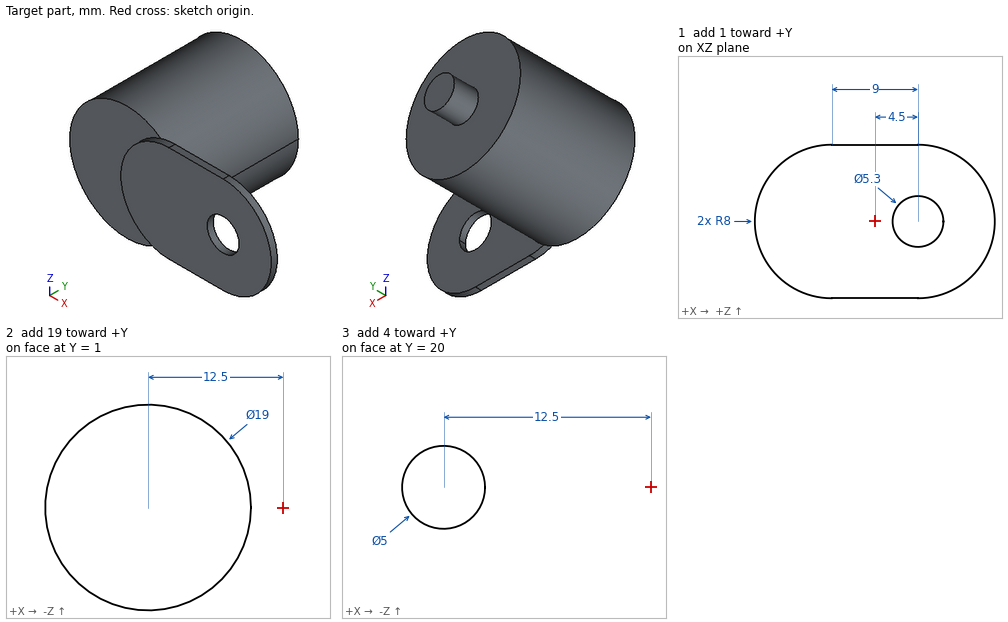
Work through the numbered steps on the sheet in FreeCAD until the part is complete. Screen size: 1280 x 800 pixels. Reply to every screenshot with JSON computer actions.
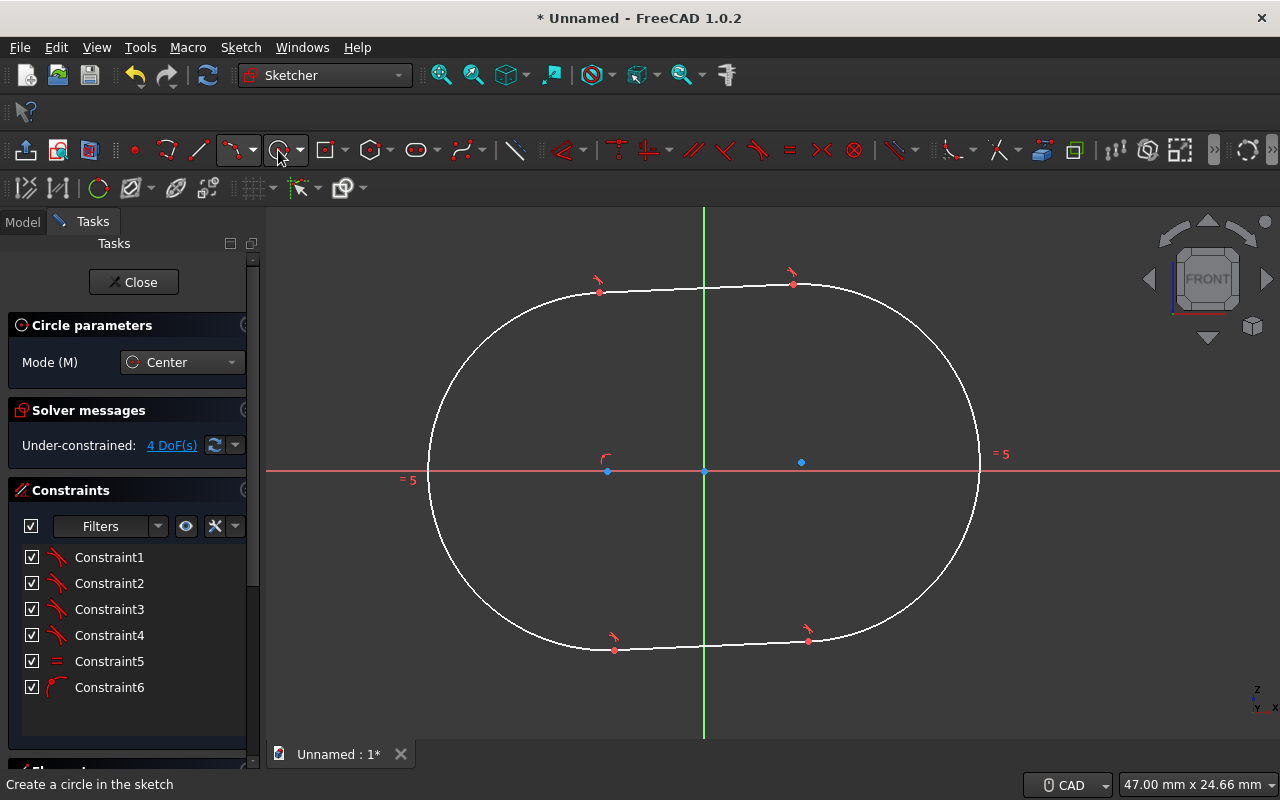
{"action": "left_click", "coordinate": [801, 463]}
{"action": "left_click", "coordinate": [842, 431]}
{"action": "key", "text": "Escape"}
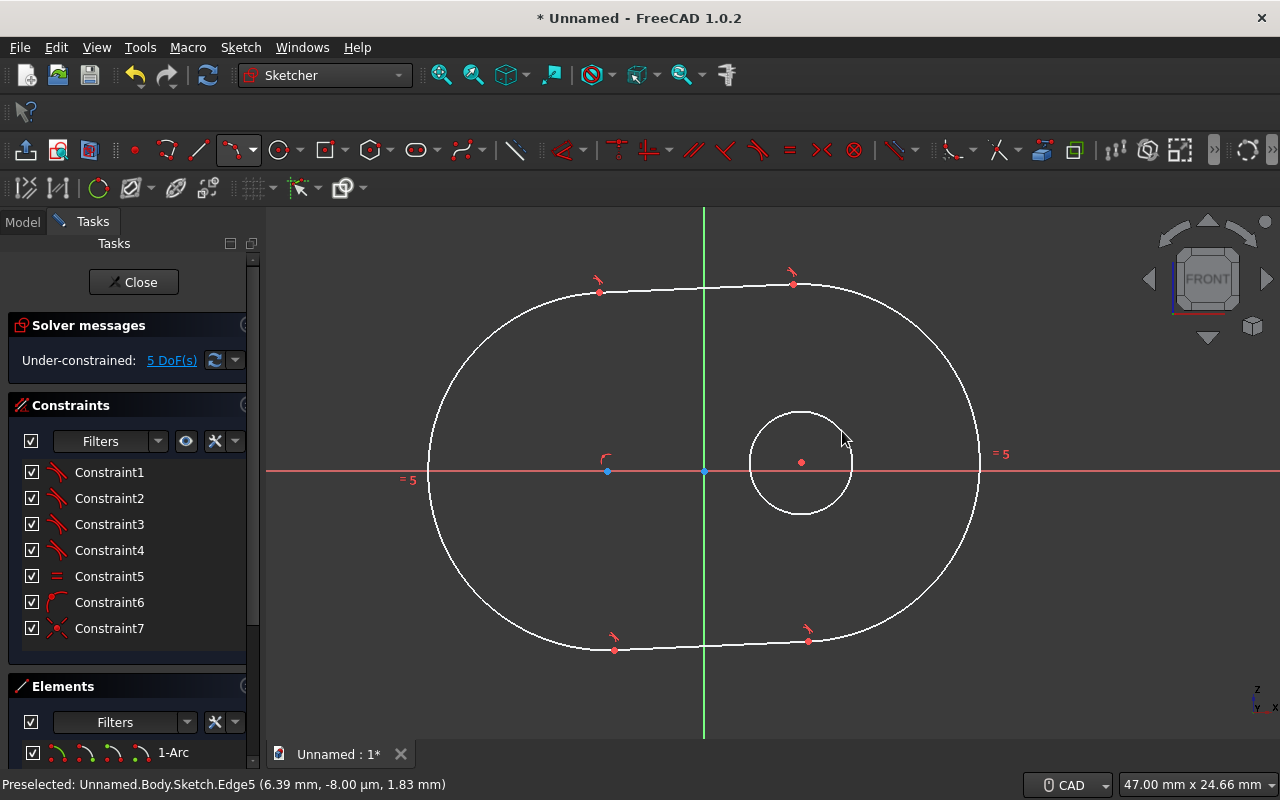
{"action": "left_click", "coordinate": [657, 290]}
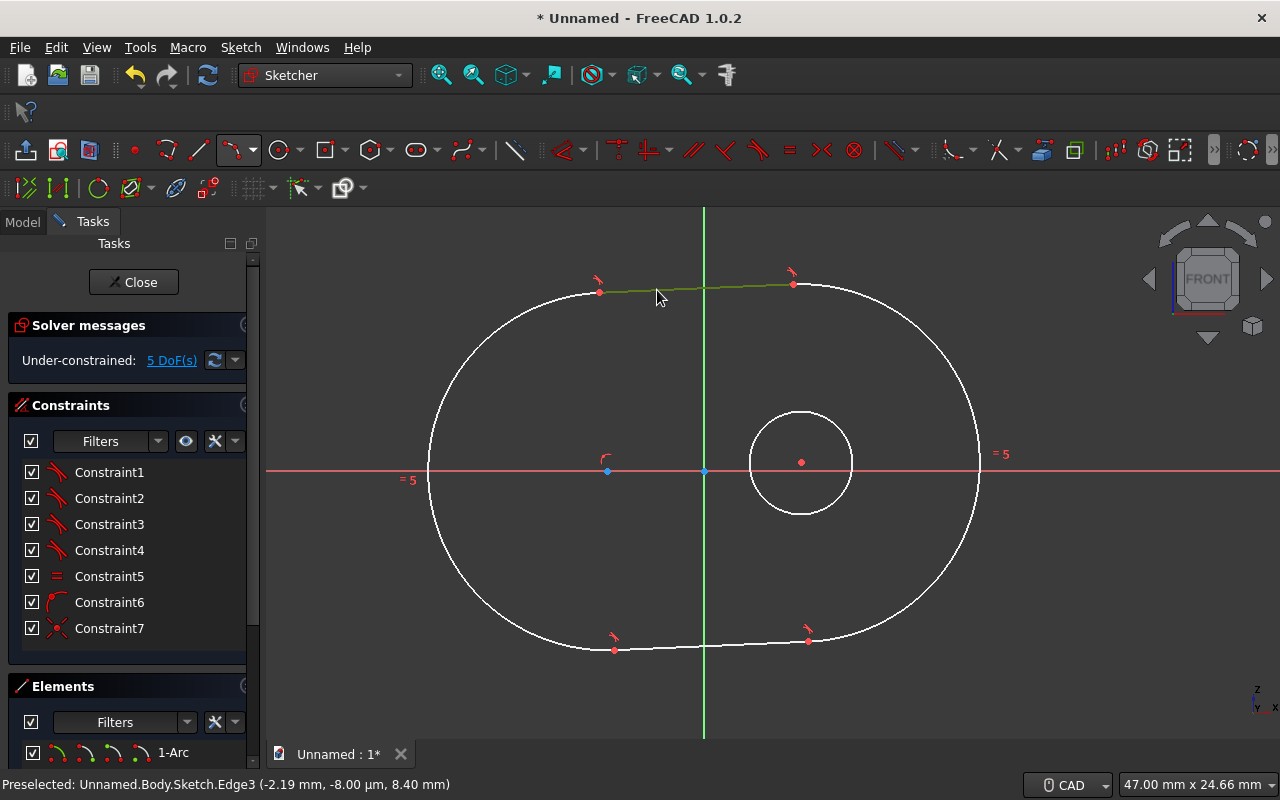
{"action": "key", "text": "h"}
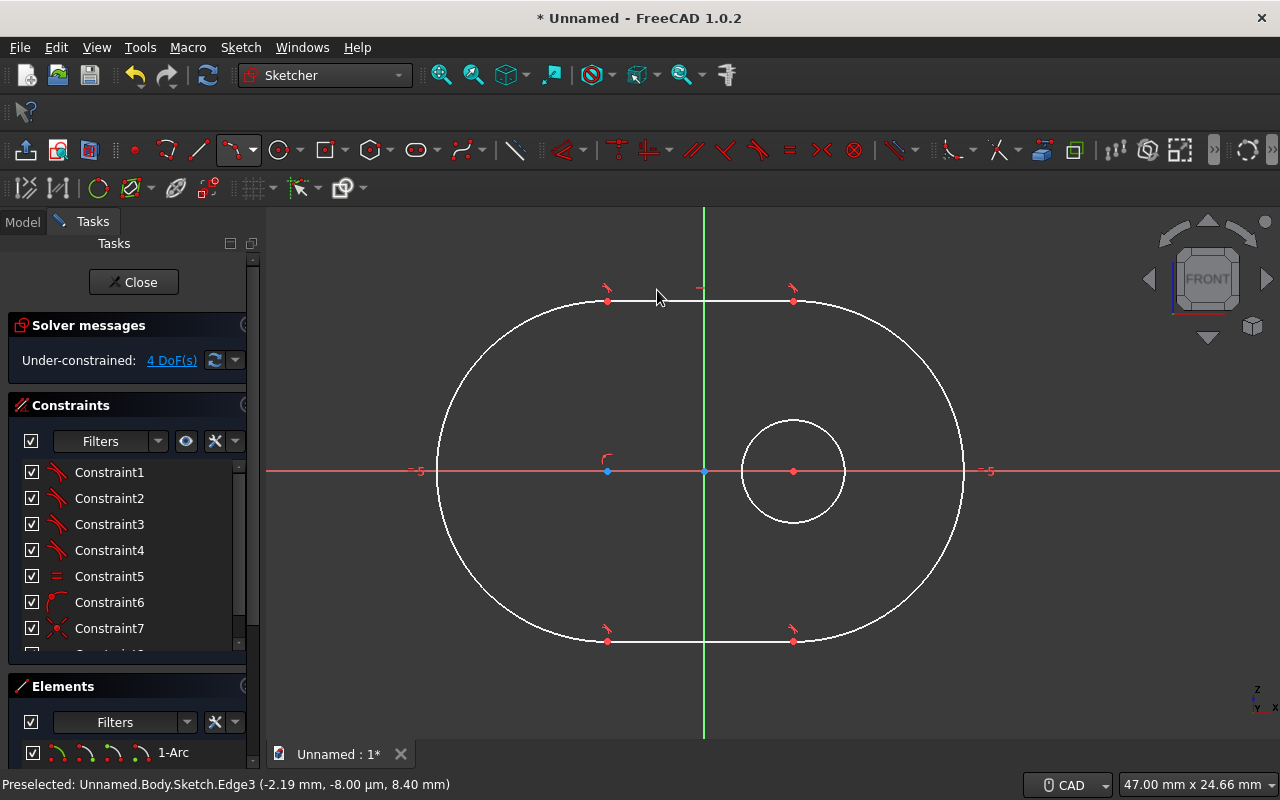
{"action": "left_click", "coordinate": [562, 150]}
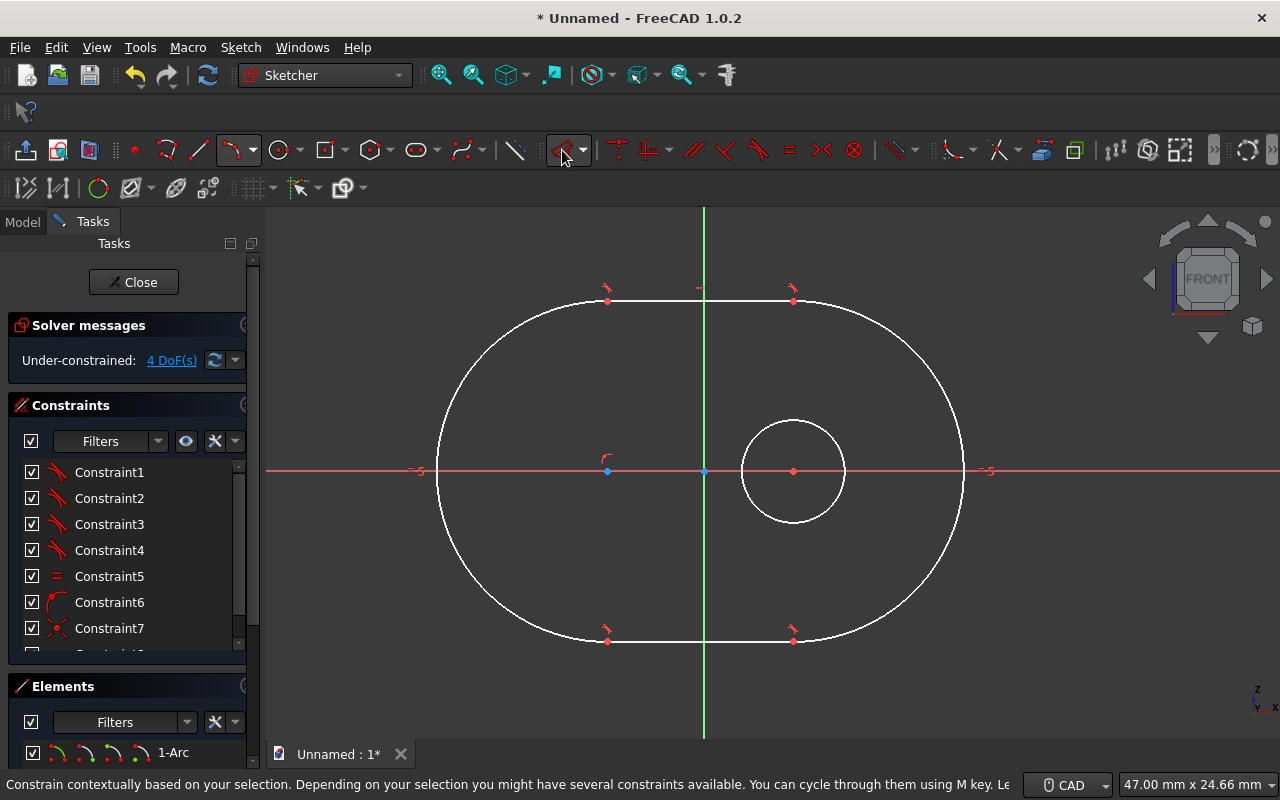
{"action": "left_click", "coordinate": [469, 371]}
{"action": "left_click", "coordinate": [443, 352]}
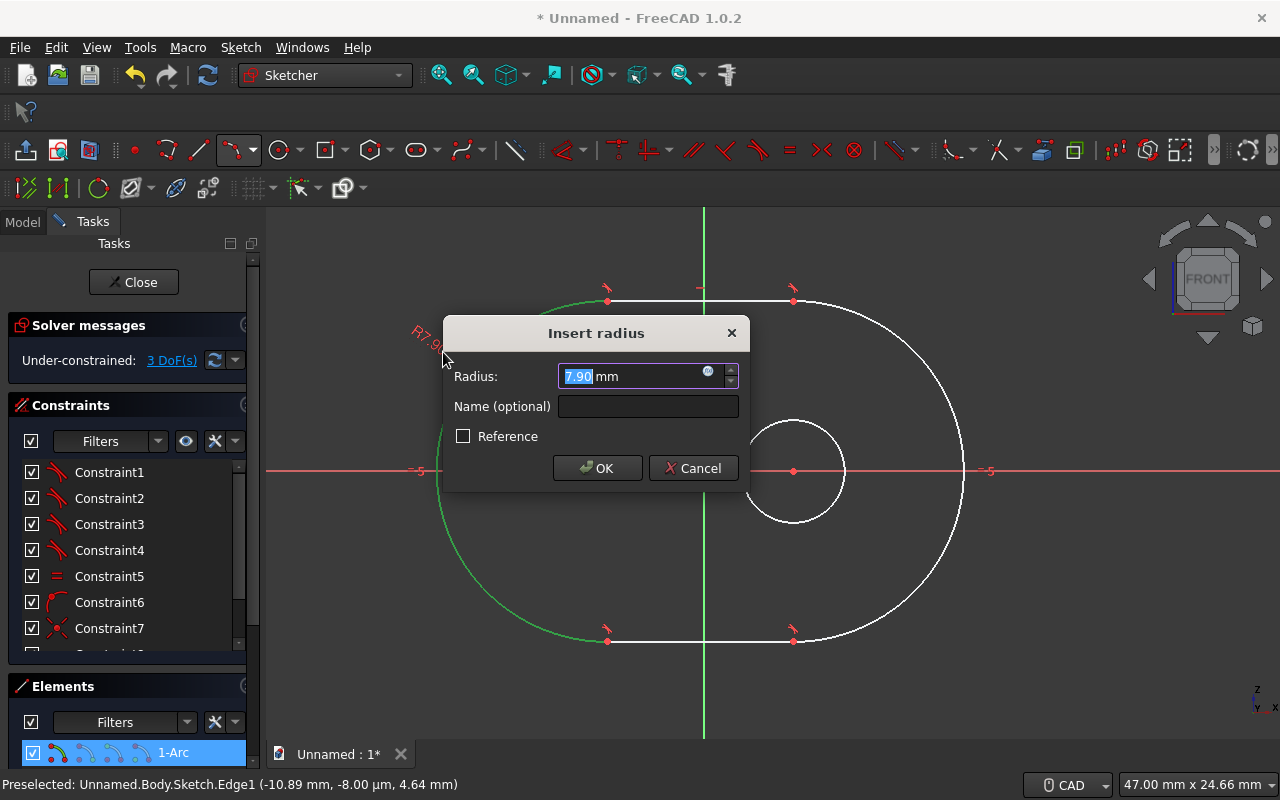
{"action": "type", "text": "8"}
{"action": "key", "text": "Return"}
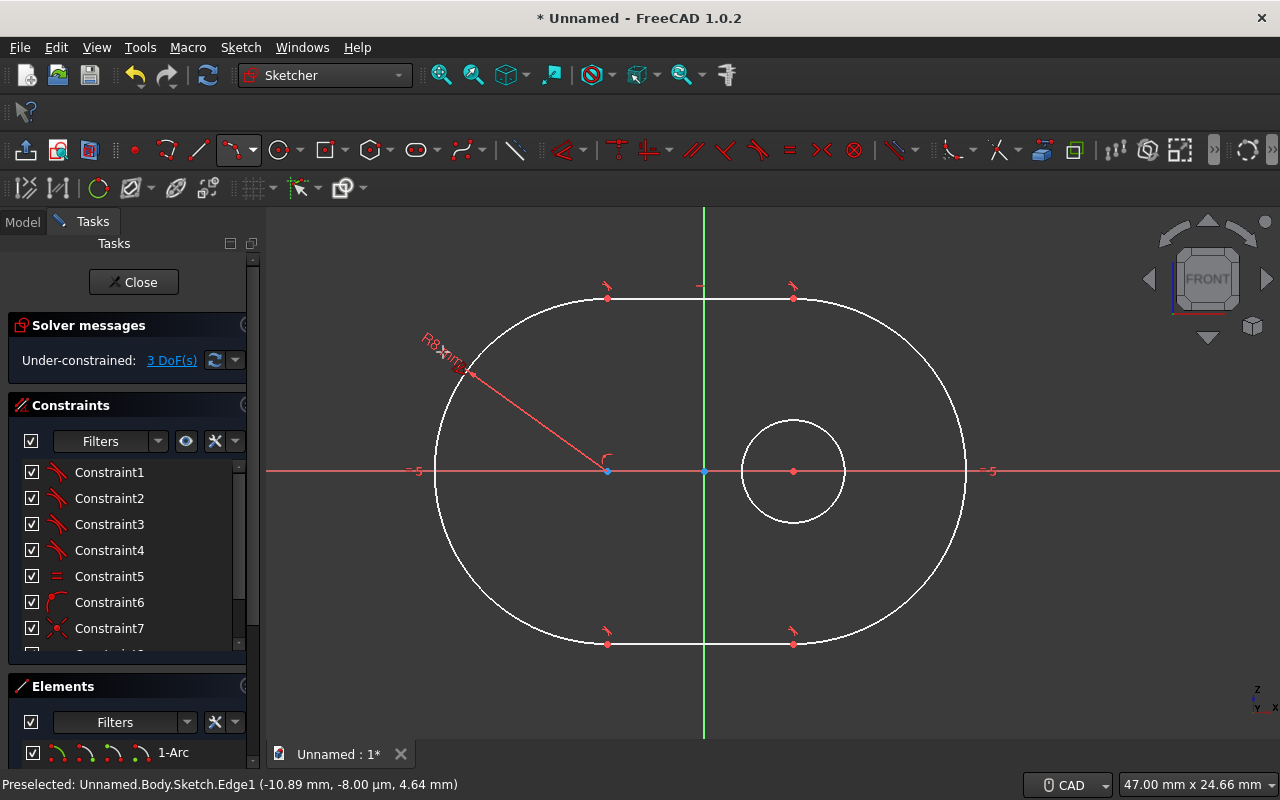
{"action": "left_click", "coordinate": [830, 435]}
{"action": "left_click", "coordinate": [853, 412]}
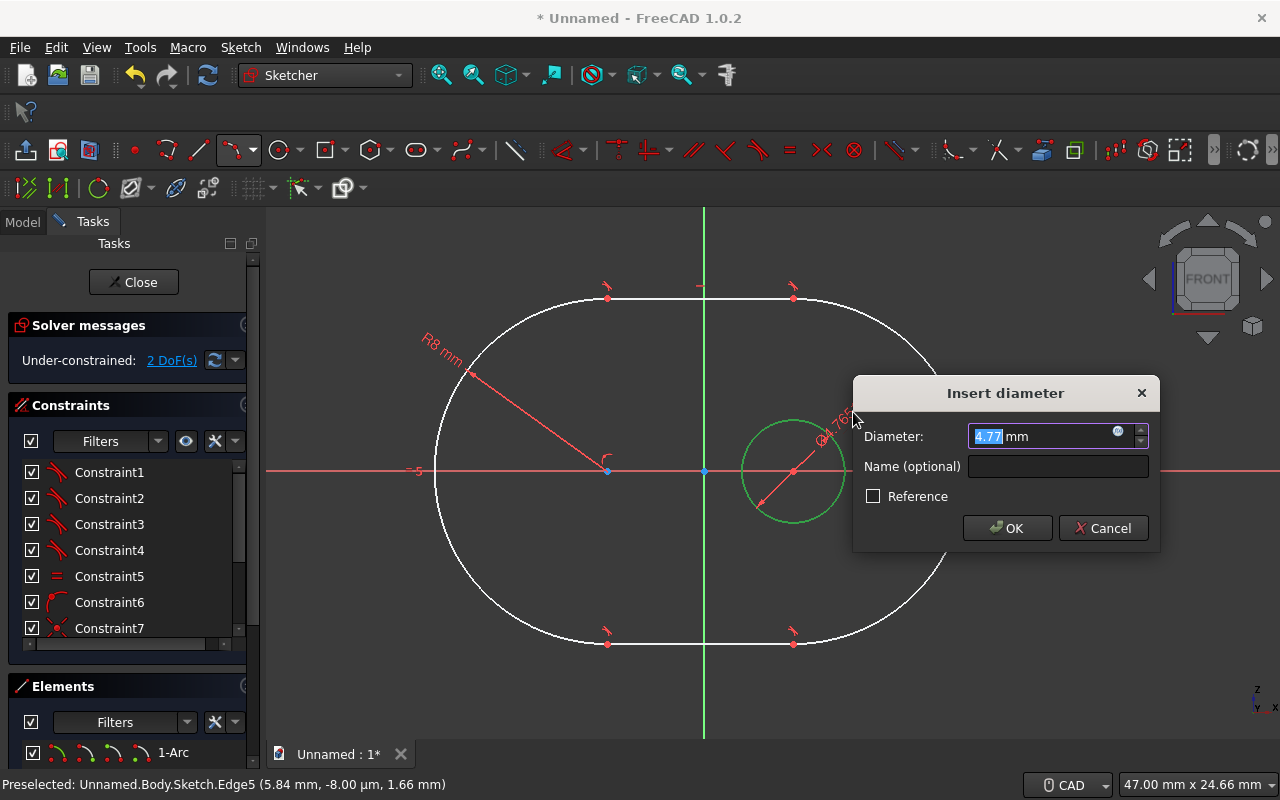
{"action": "type", "text": "5.3"}
{"action": "key", "text": "Return"}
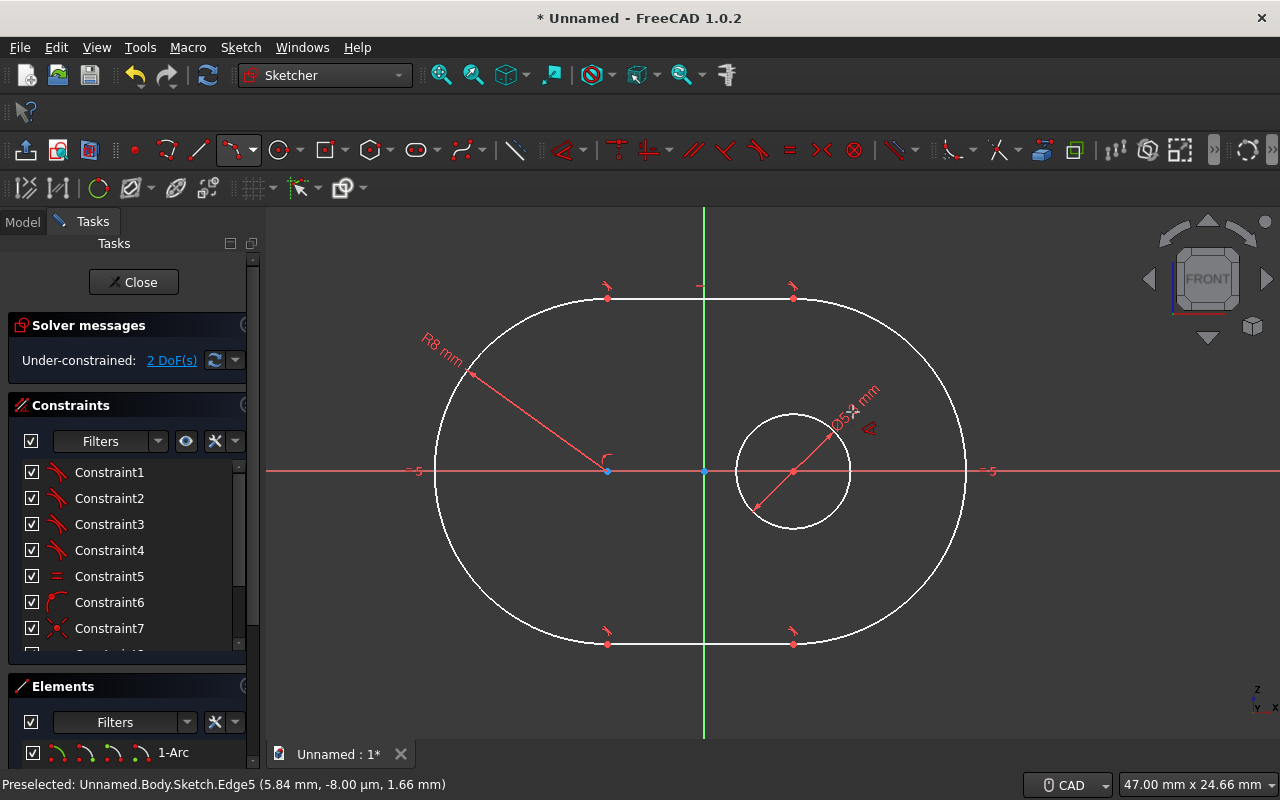
{"action": "left_click", "coordinate": [663, 299]}
{"action": "left_click", "coordinate": [657, 265]}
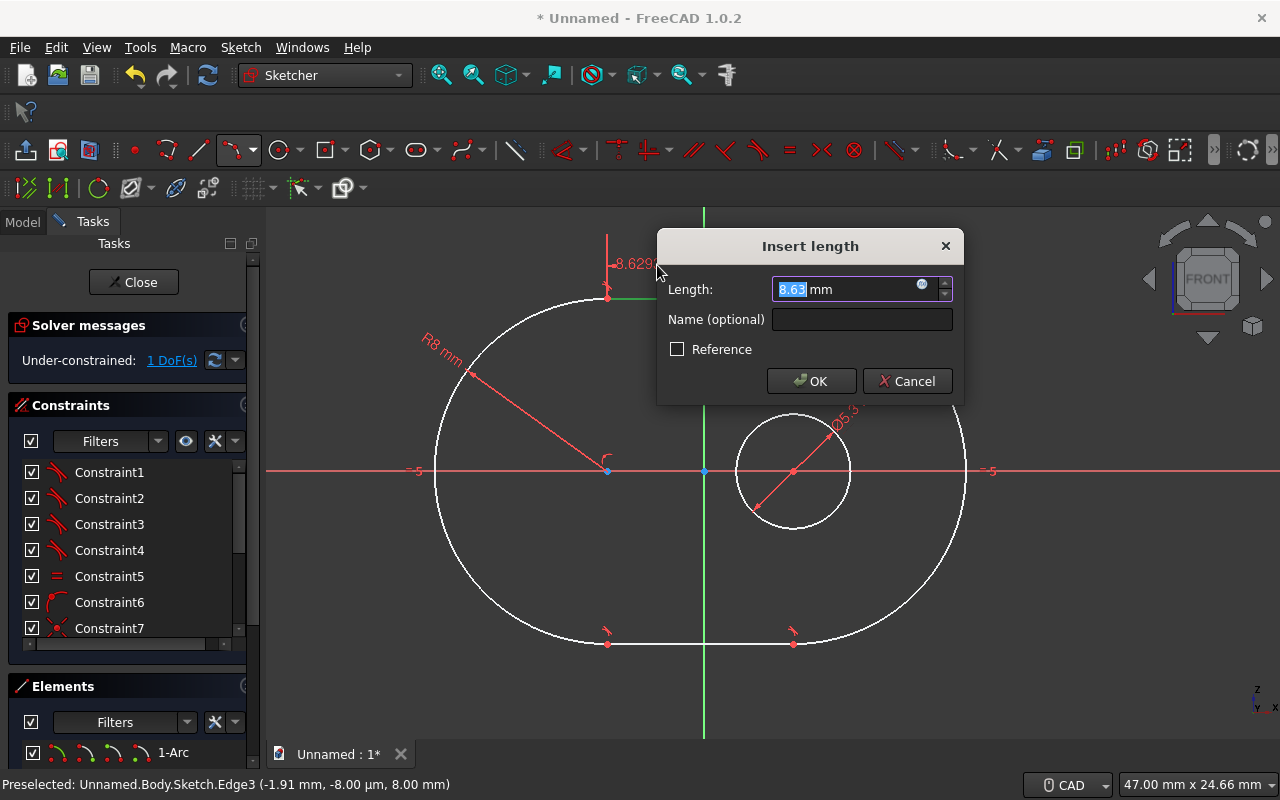
{"action": "type", "text": "9"}
{"action": "key", "text": "Return"}